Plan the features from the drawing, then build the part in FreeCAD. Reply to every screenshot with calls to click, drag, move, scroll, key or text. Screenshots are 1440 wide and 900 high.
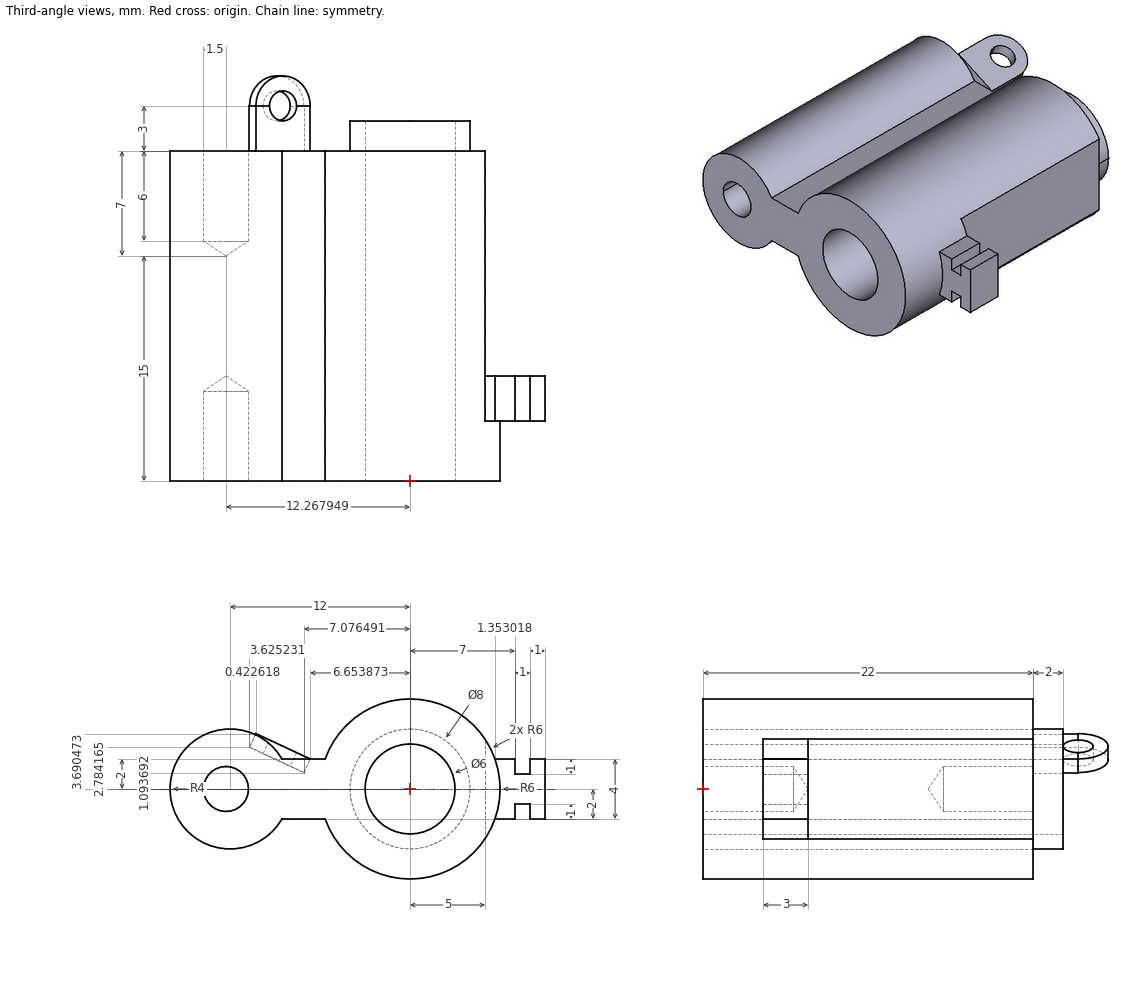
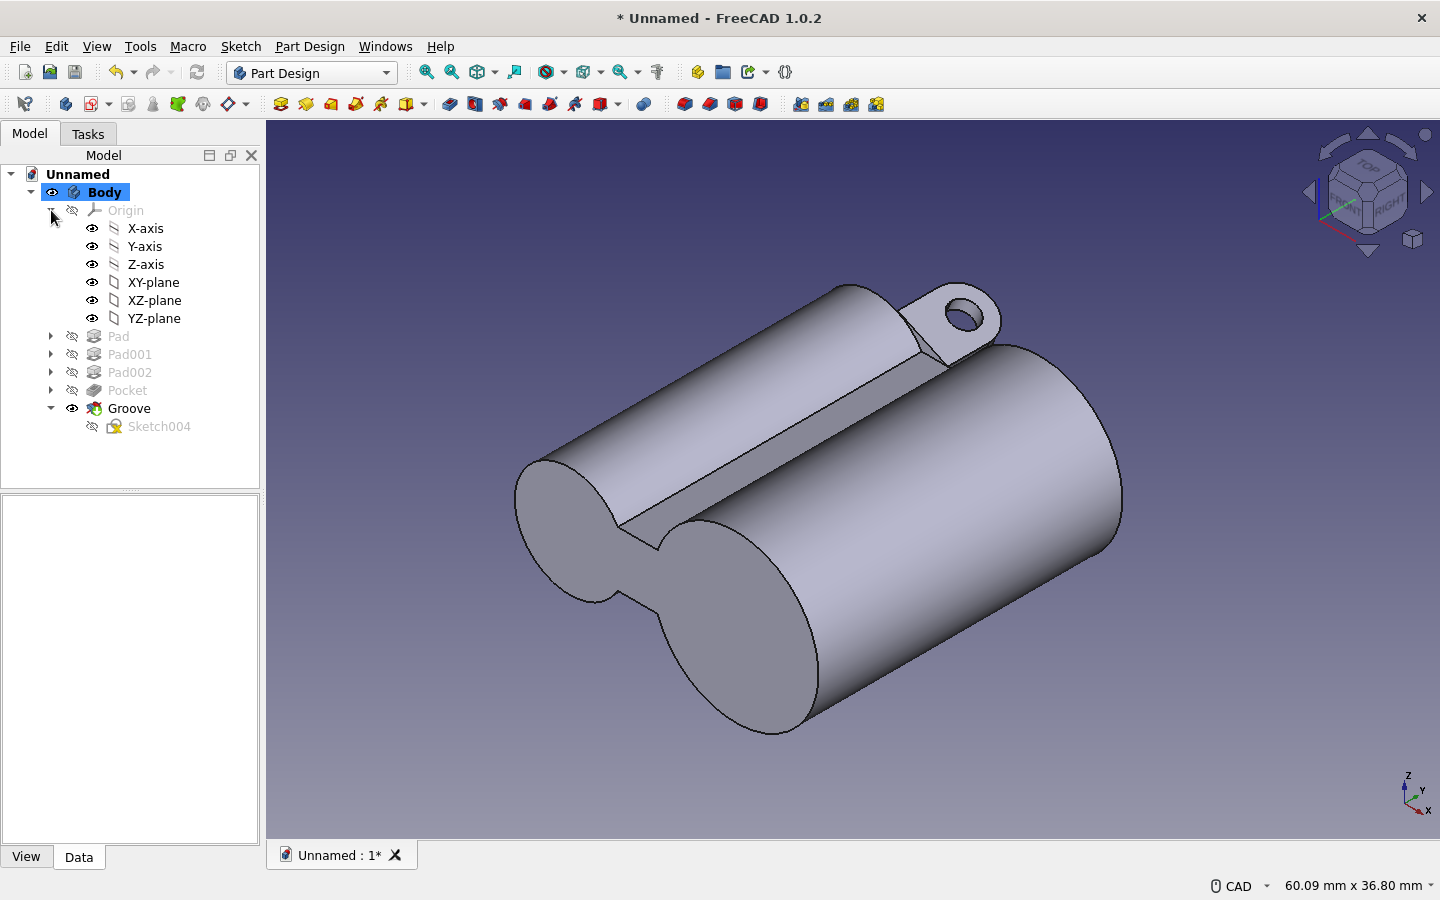
click(137, 300)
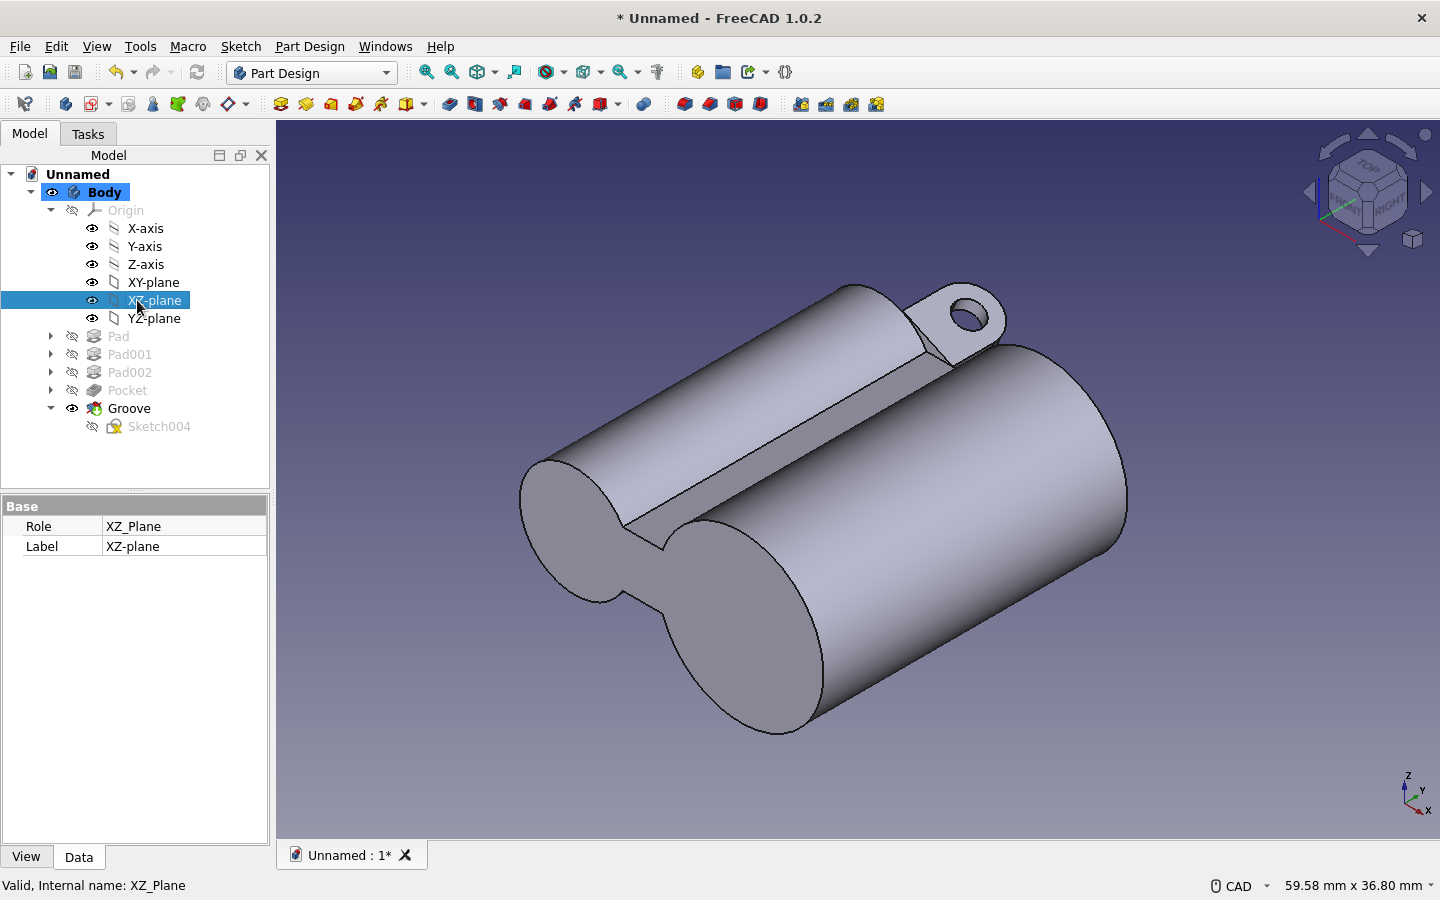
click(228, 104)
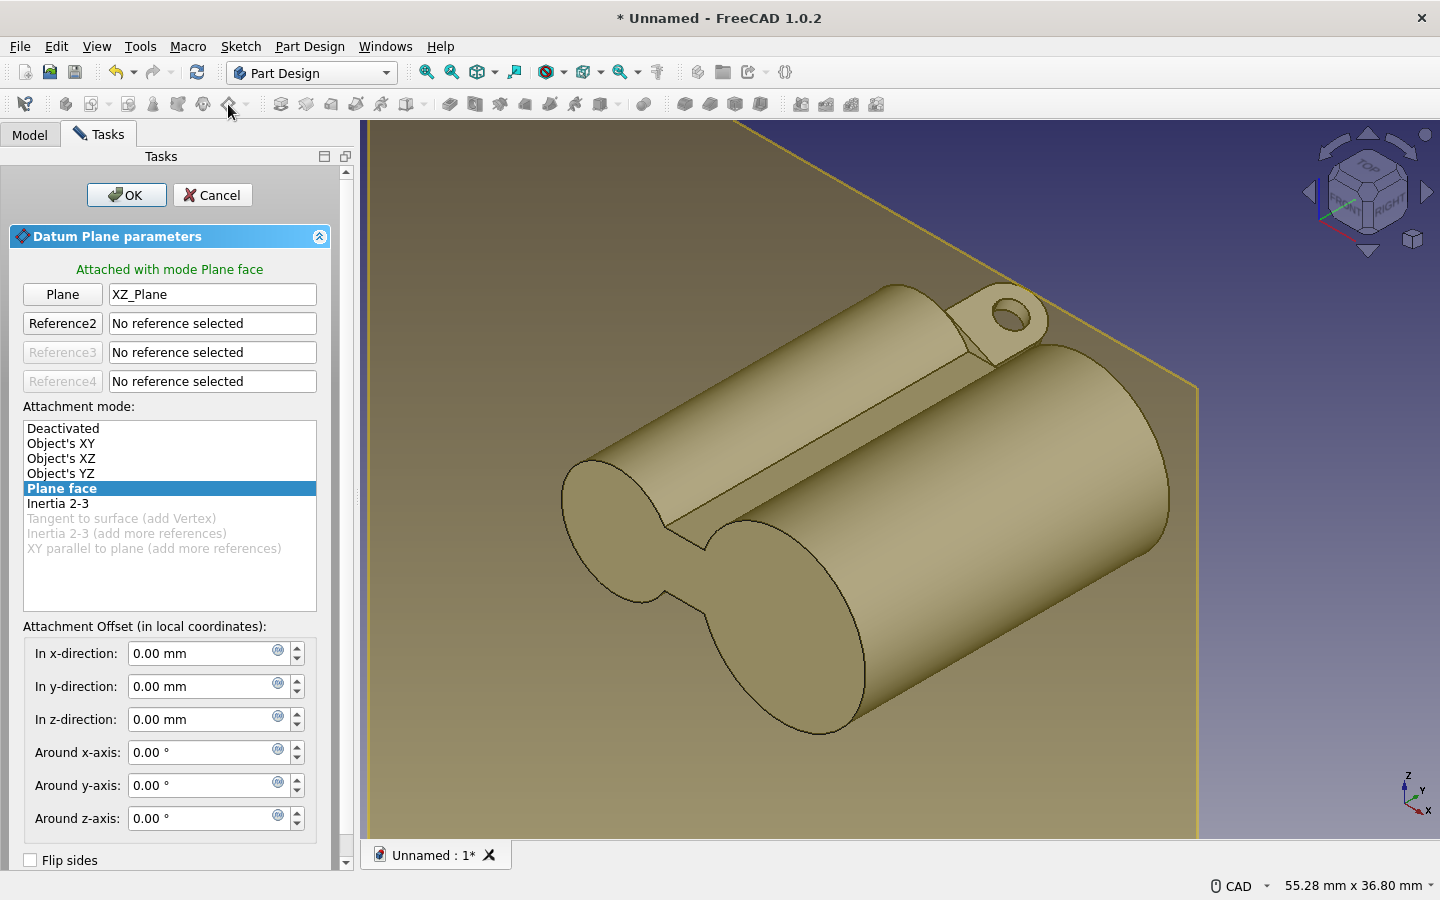
triple_click(210, 720)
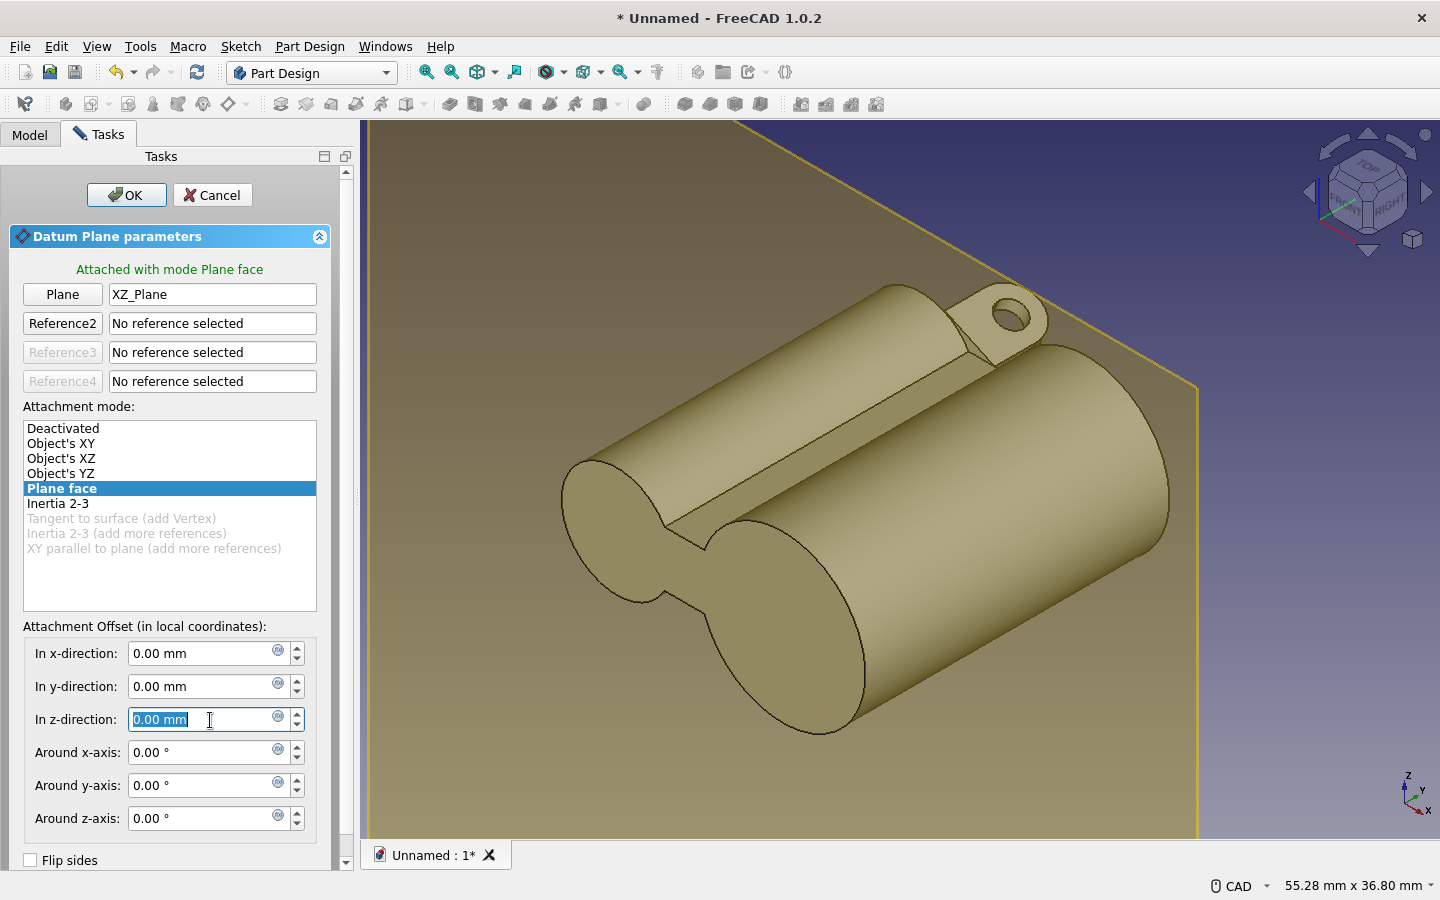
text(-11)
key(Tab)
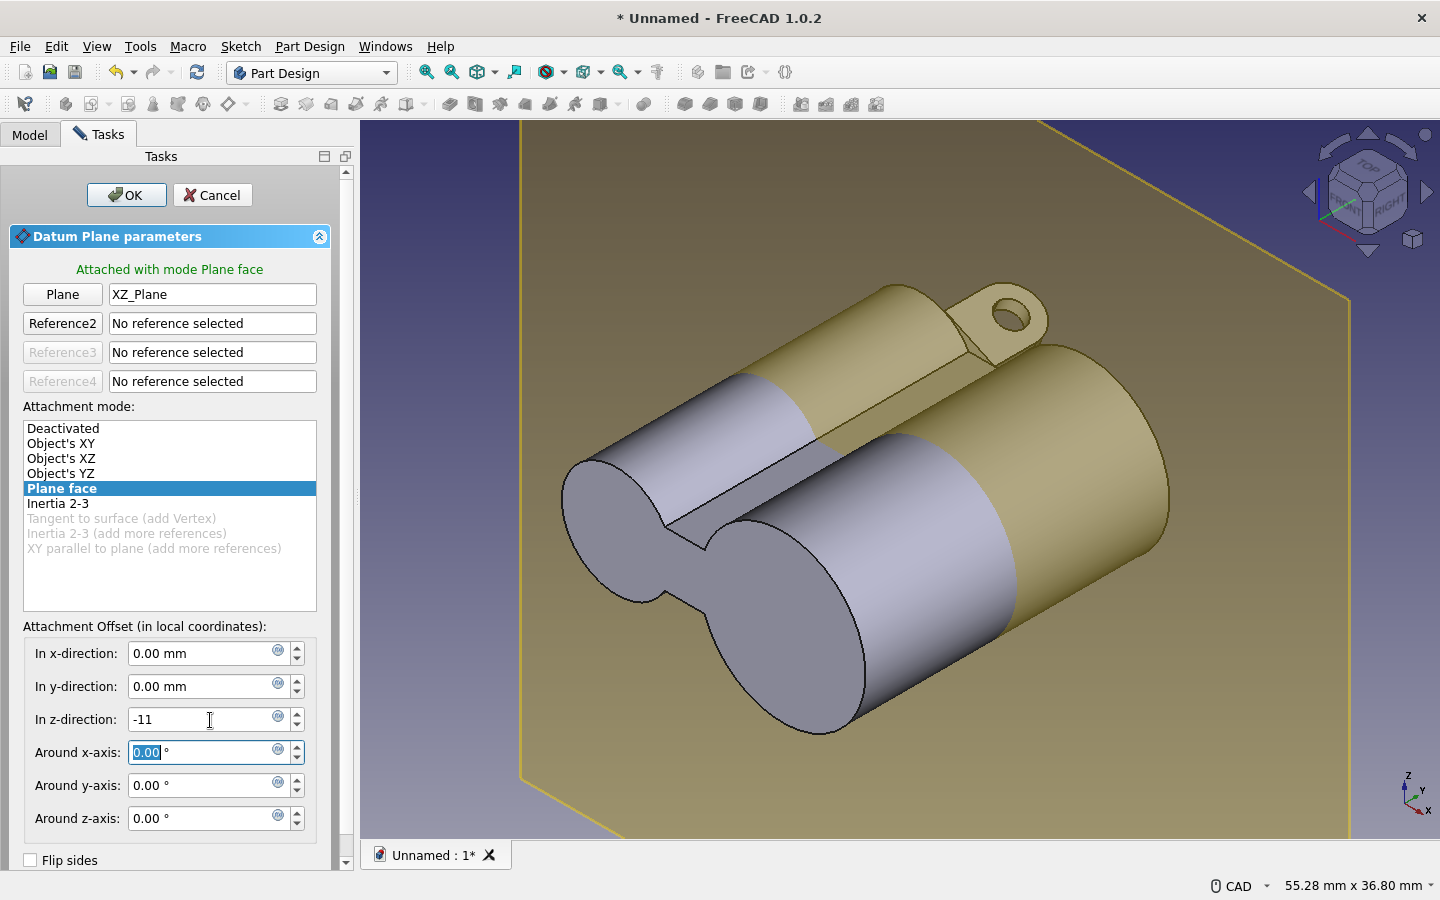
click(127, 195)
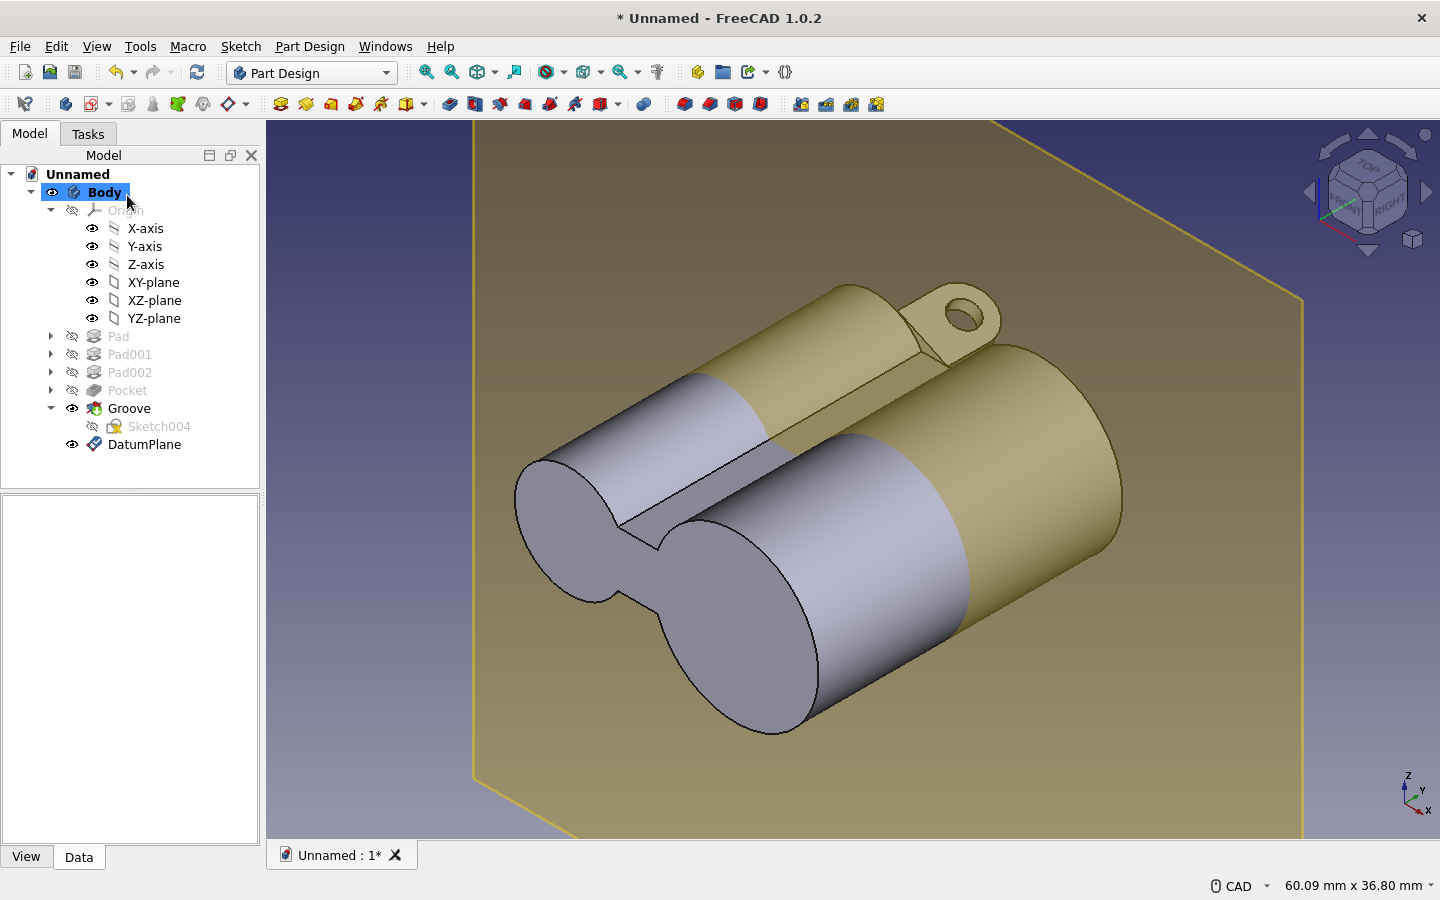
click(117, 408)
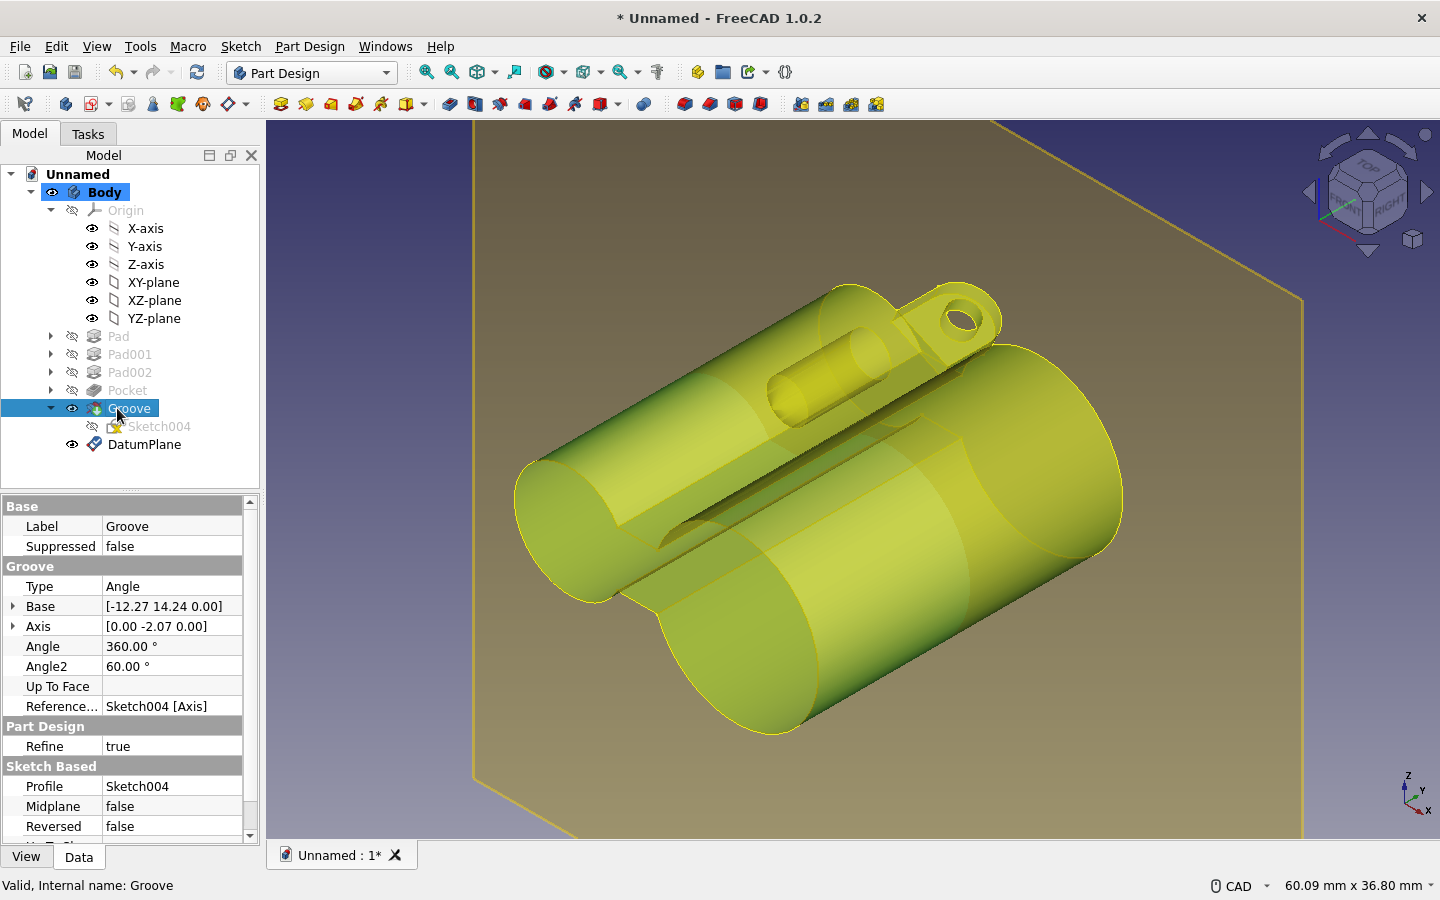
click(801, 104)